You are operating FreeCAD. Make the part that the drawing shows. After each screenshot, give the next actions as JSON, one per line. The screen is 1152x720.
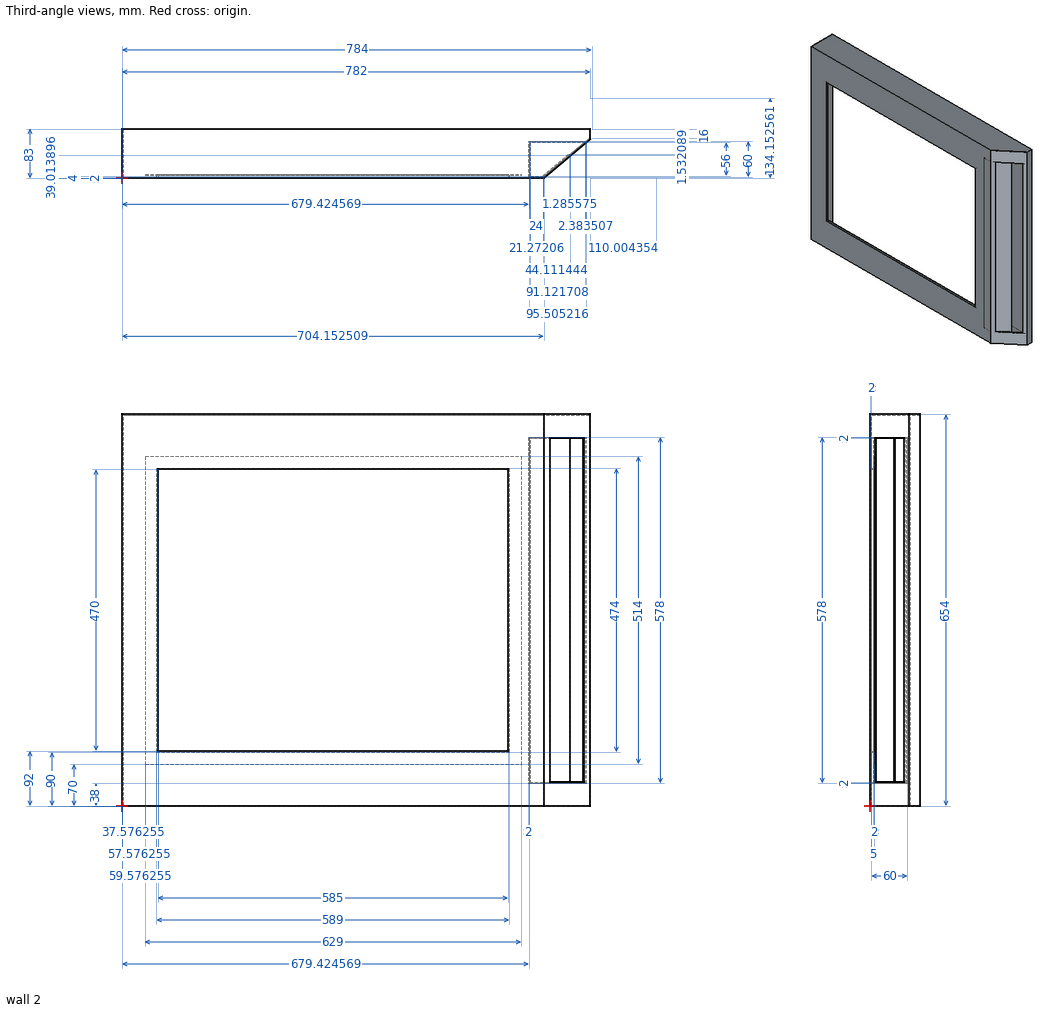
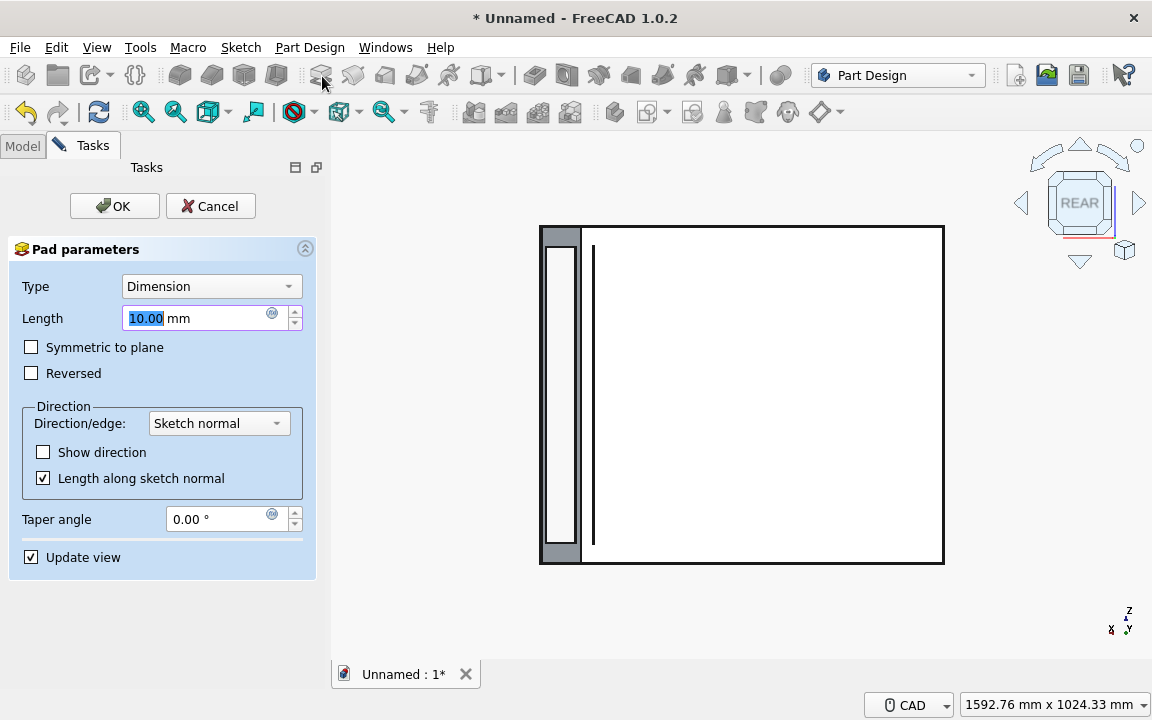
{"action": "type", "text": "60"}
{"action": "key", "text": "Tab"}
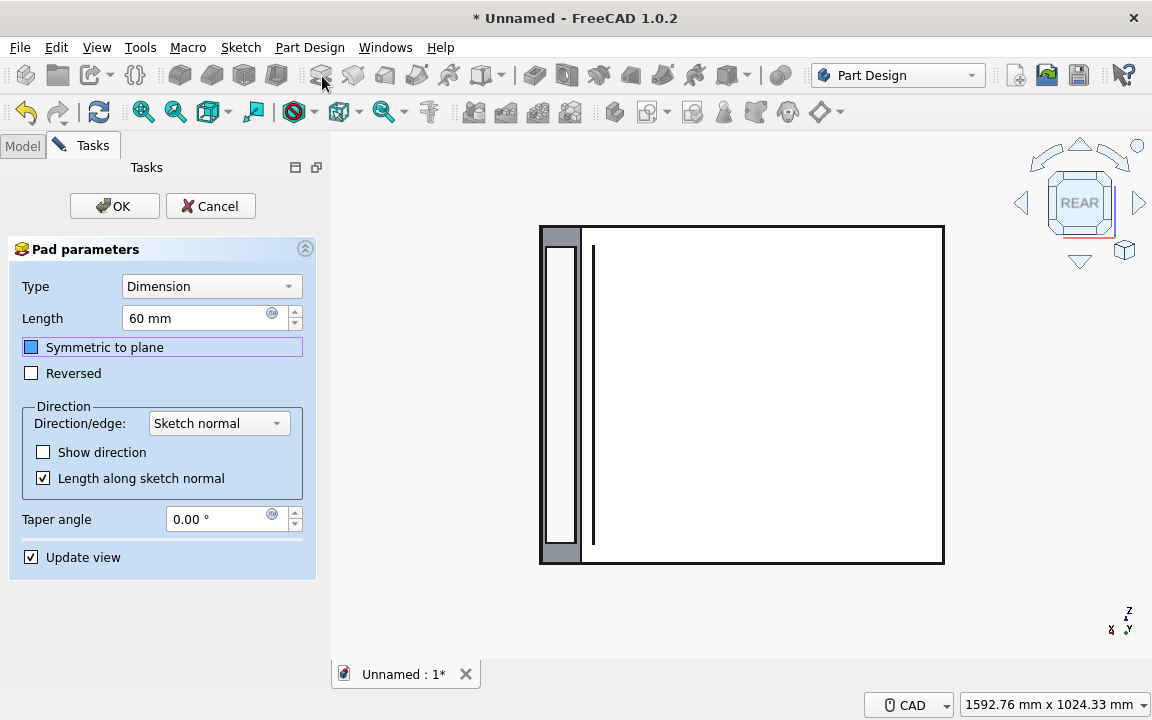
{"action": "left_click", "coordinate": [115, 206]}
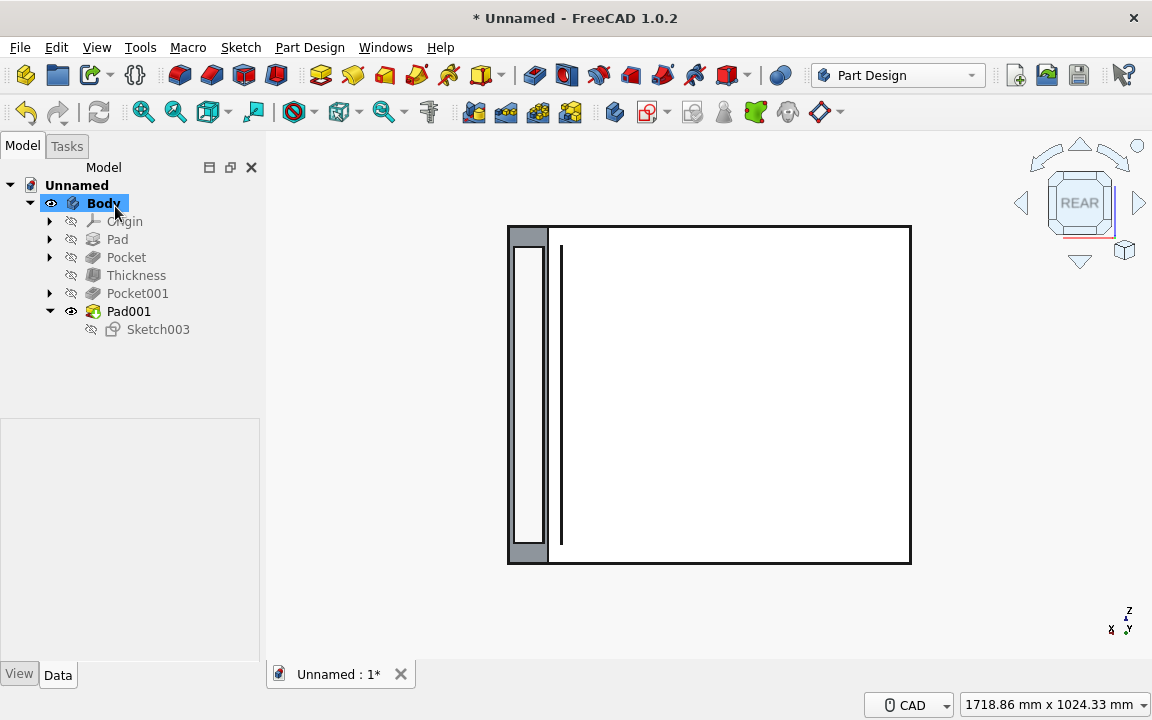
{"action": "key", "text": "0"}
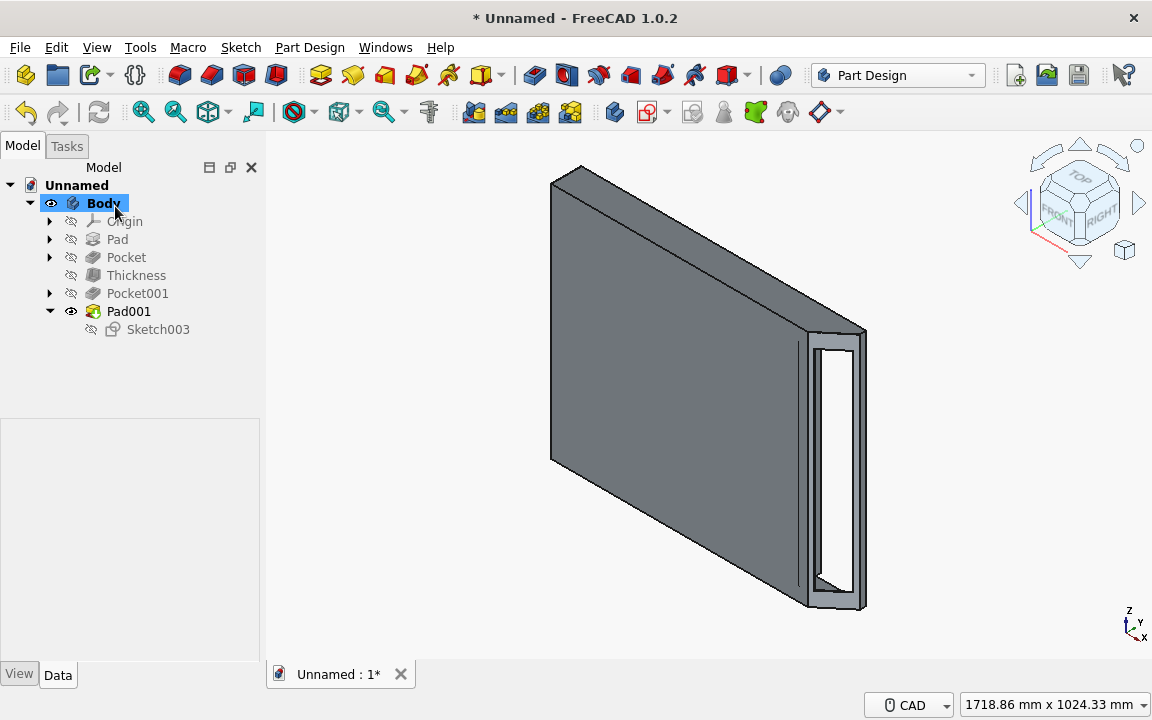
{"action": "left_click", "coordinate": [679, 394]}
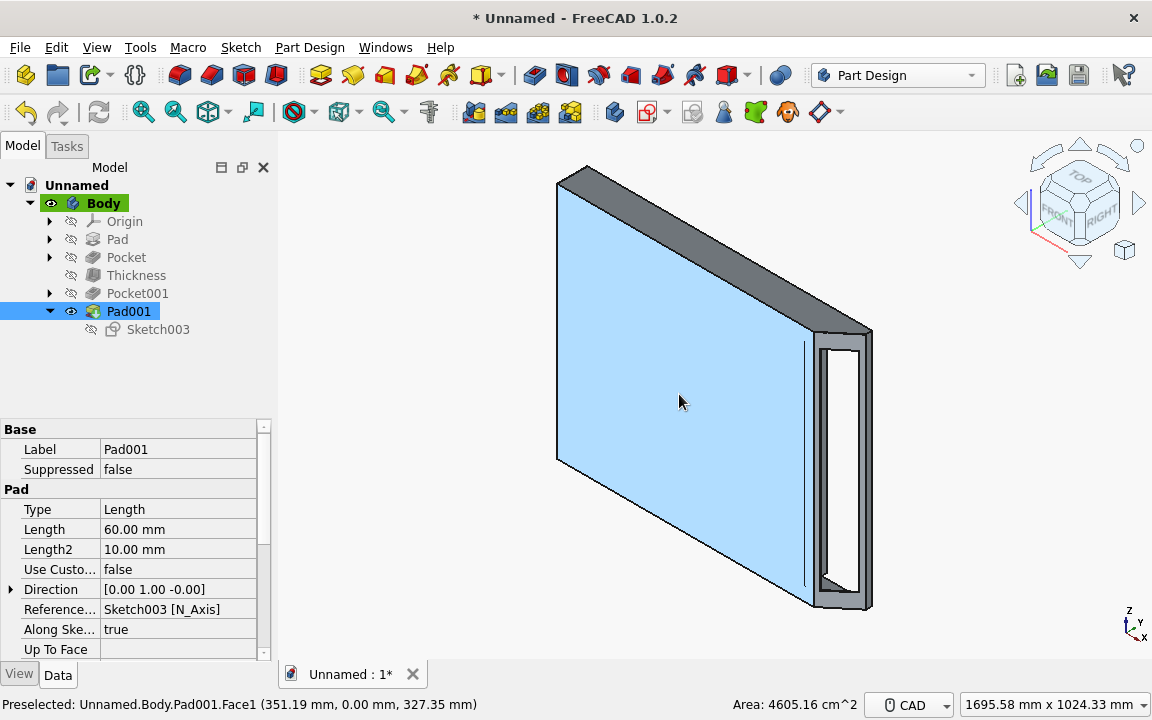
{"action": "left_click", "coordinate": [648, 112]}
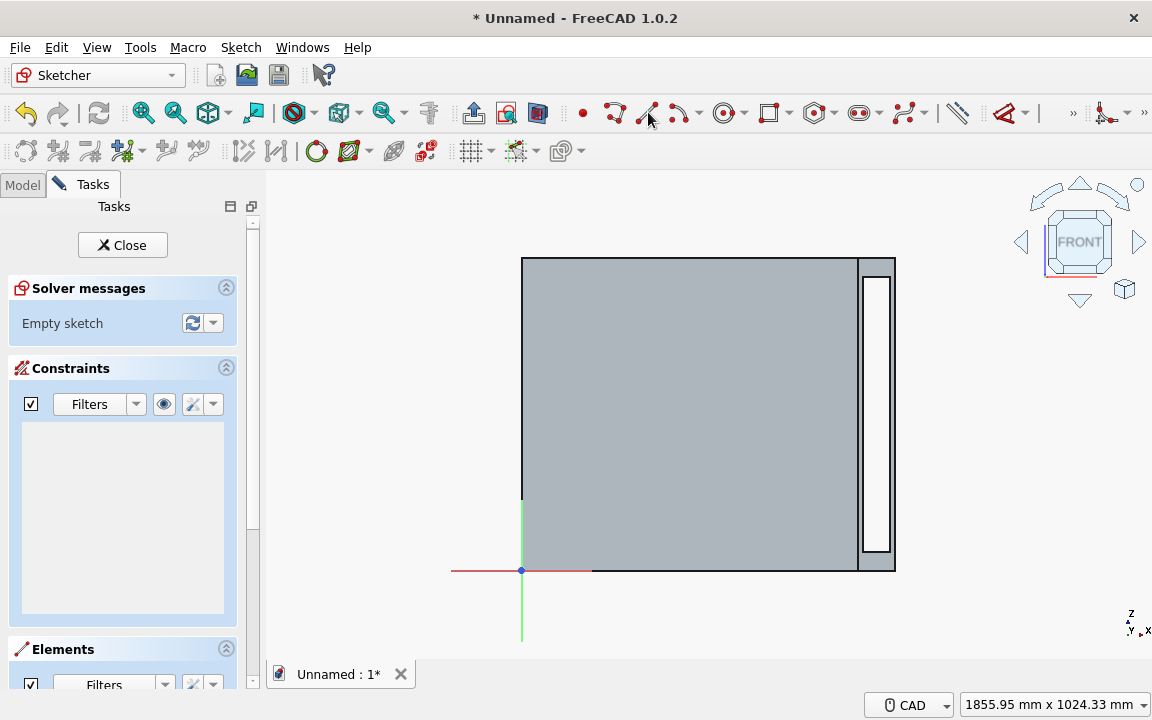
{"action": "key", "text": "g r"}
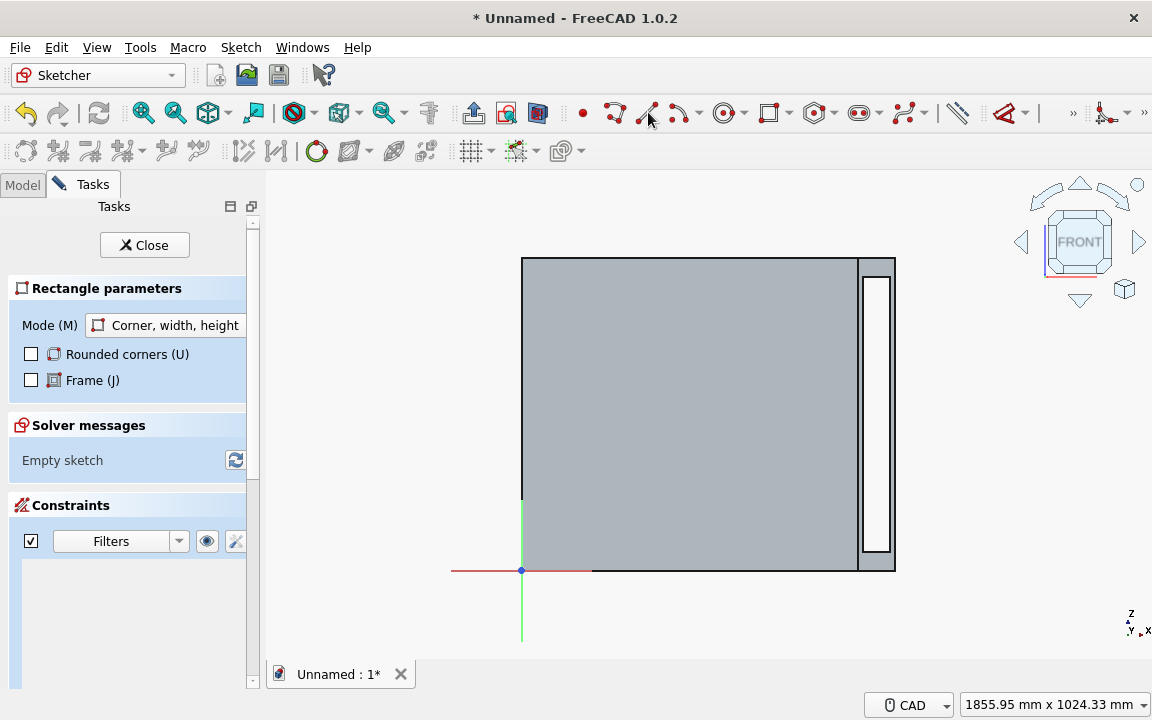
{"action": "left_click", "coordinate": [550, 302]}
{"action": "left_click", "coordinate": [830, 527]}
{"action": "key", "text": "Escape"}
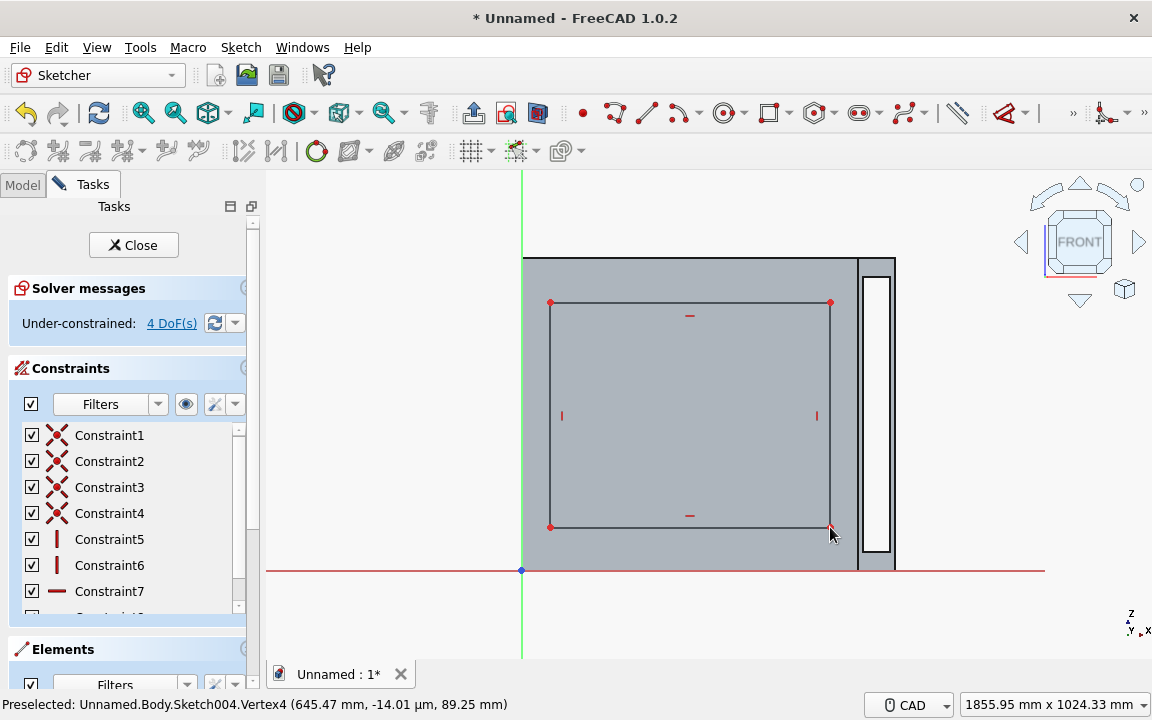
{"action": "key", "text": "d"}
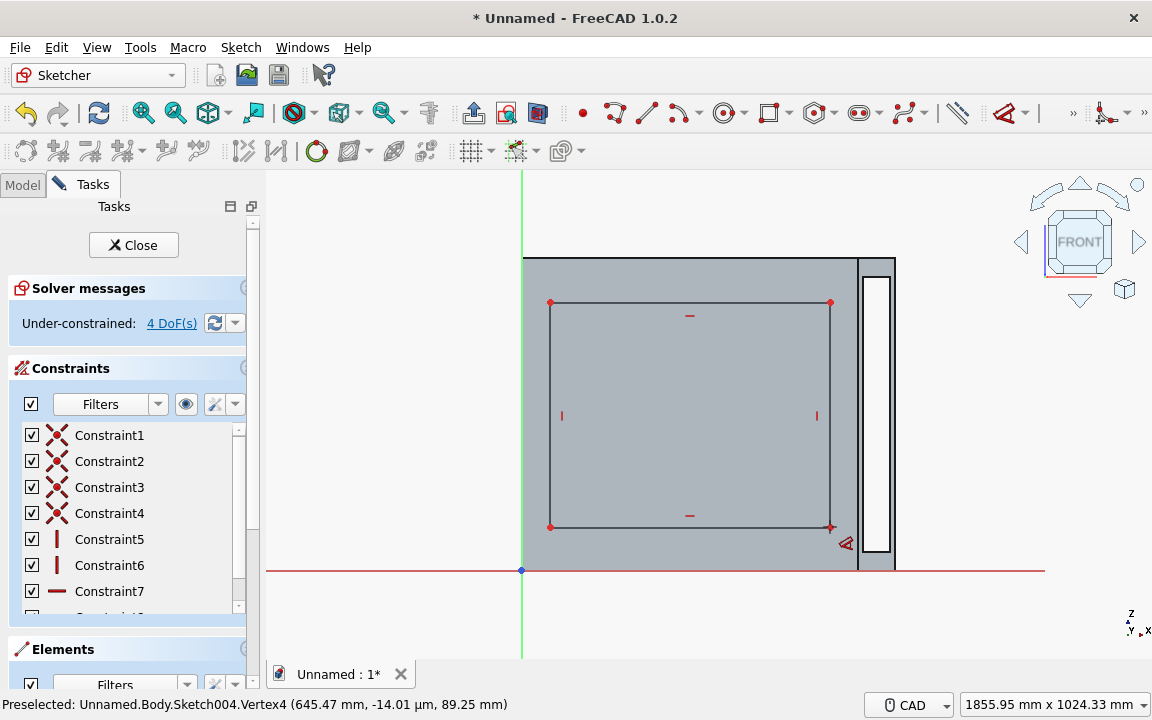
{"action": "left_click", "coordinate": [550, 370]}
{"action": "left_click", "coordinate": [584, 415]}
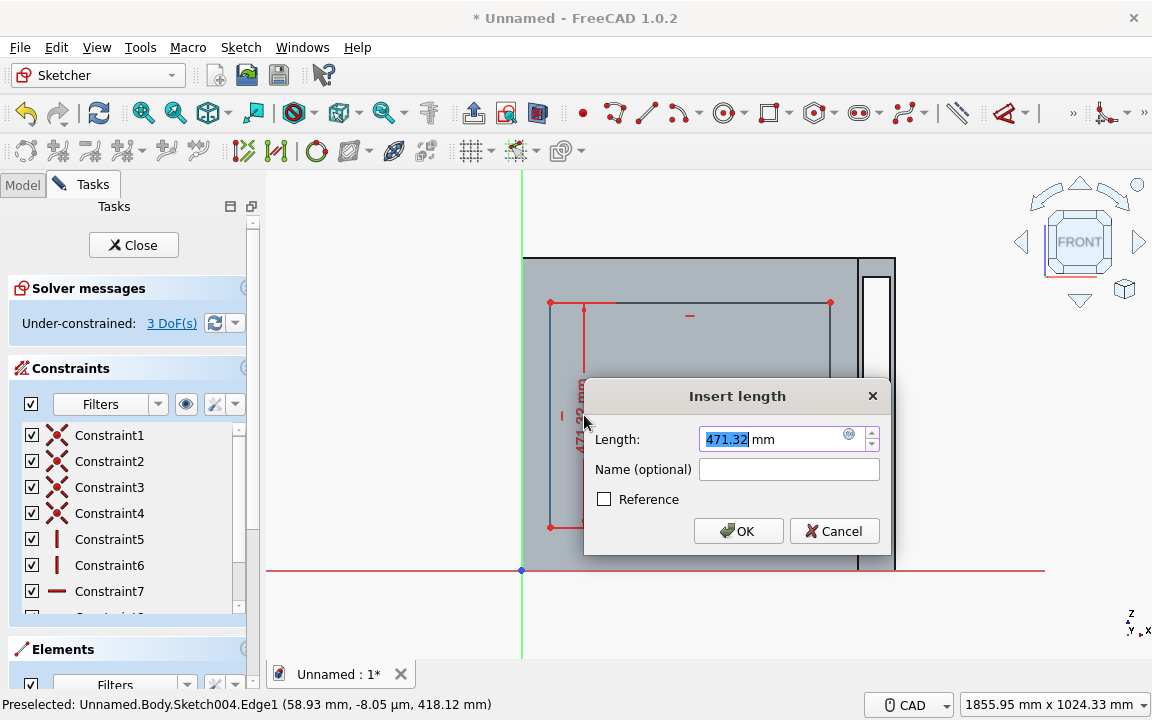
{"action": "type", "text": "470"}
{"action": "key", "text": "Return"}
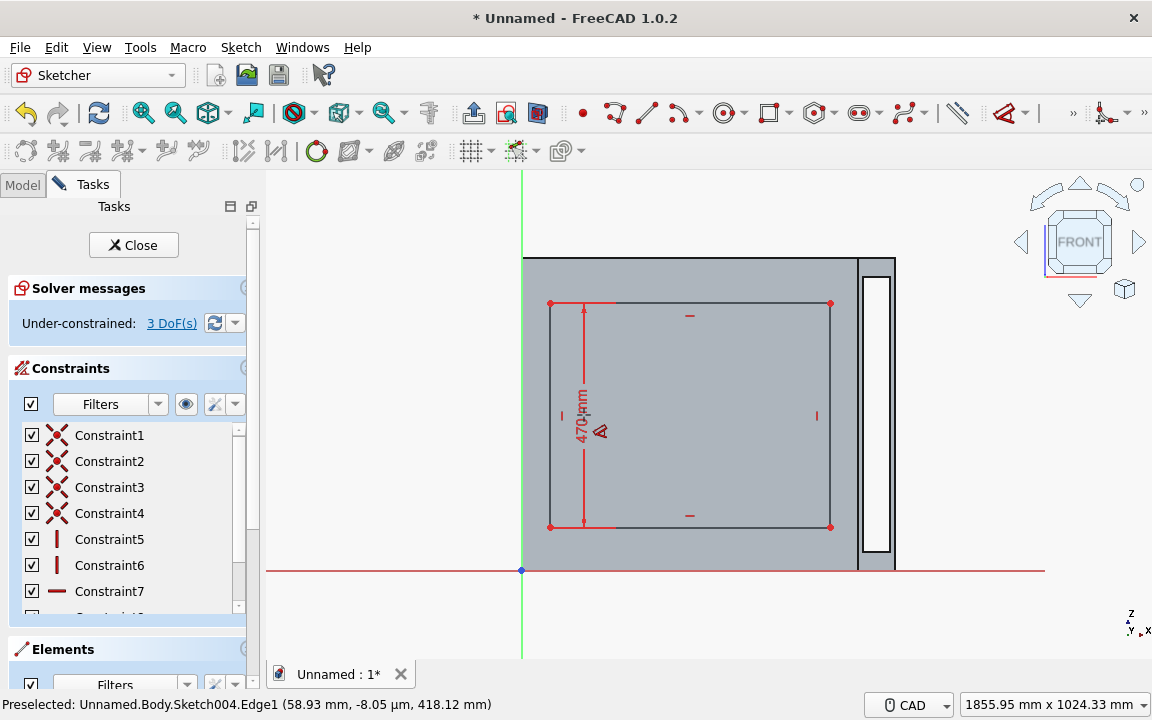
{"action": "left_click", "coordinate": [634, 528]}
{"action": "left_click", "coordinate": [690, 494]}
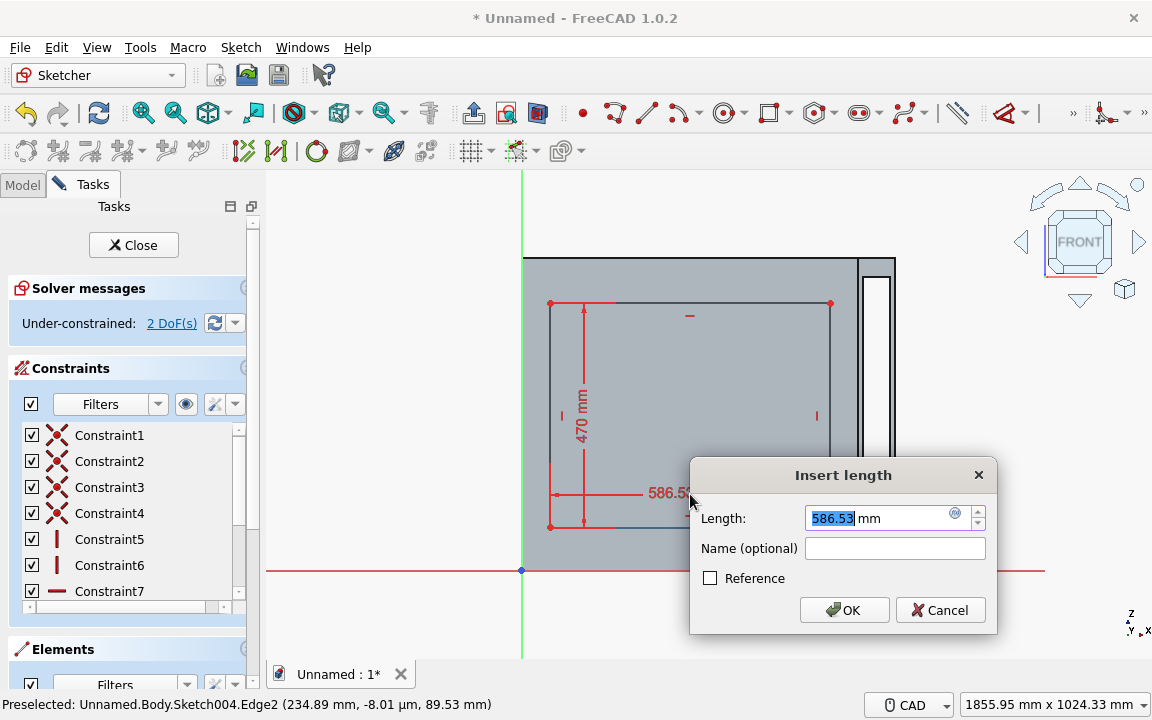
{"action": "type", "text": "585"}
{"action": "key", "text": "Return"}